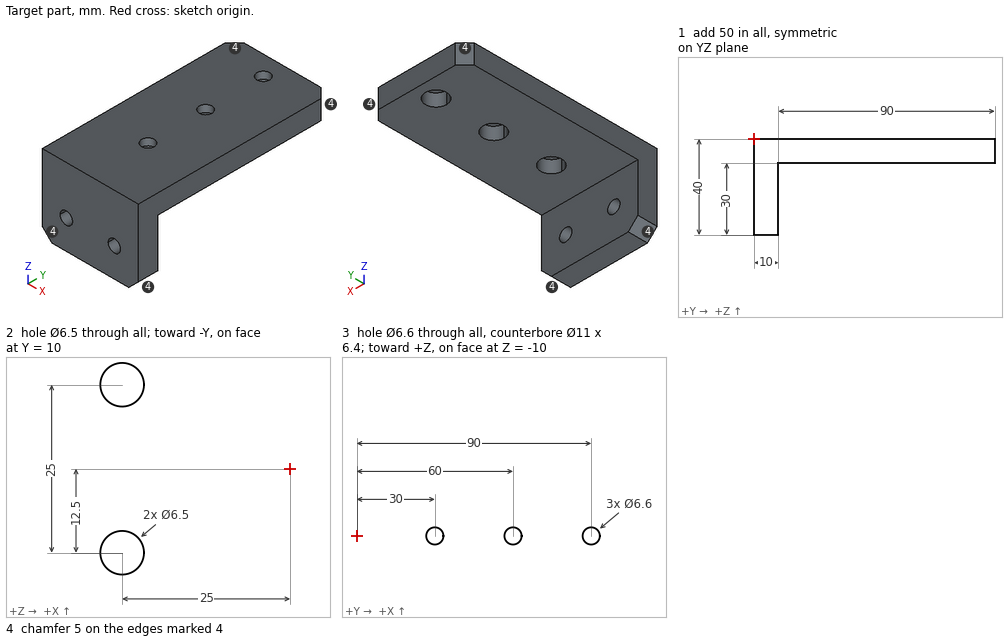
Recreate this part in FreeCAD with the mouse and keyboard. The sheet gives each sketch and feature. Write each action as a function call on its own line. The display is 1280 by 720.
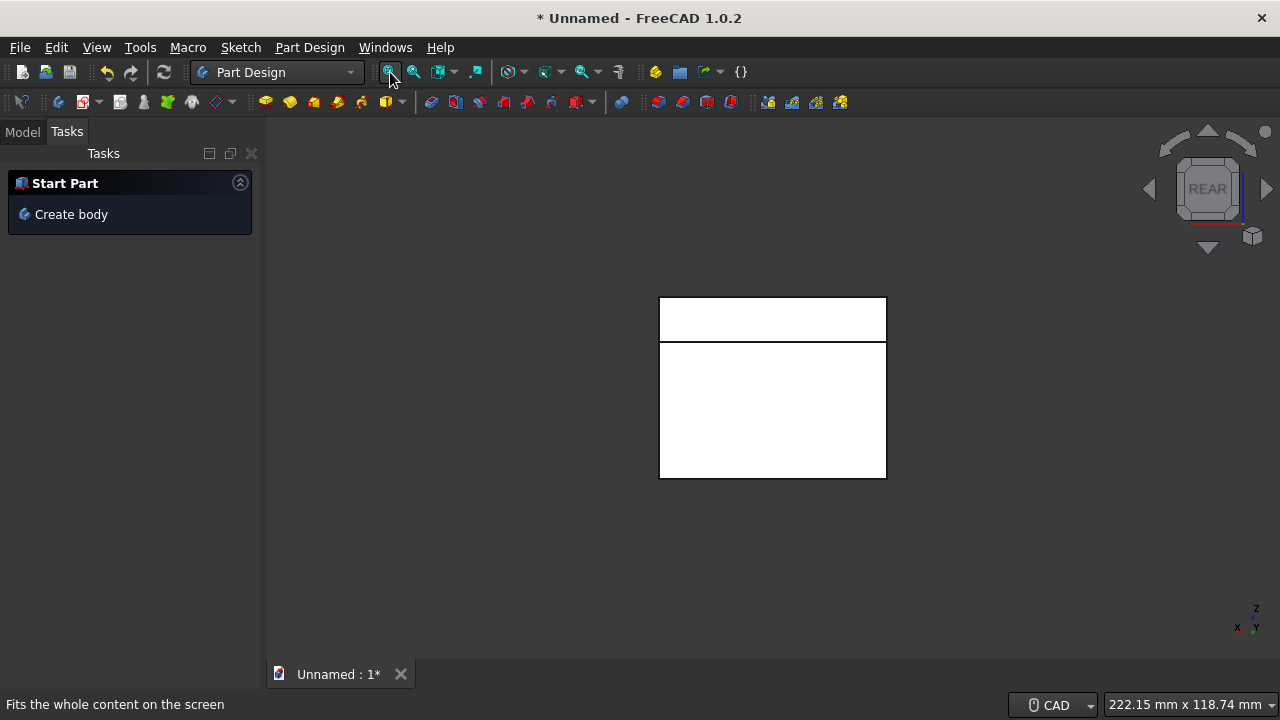
click(806, 410)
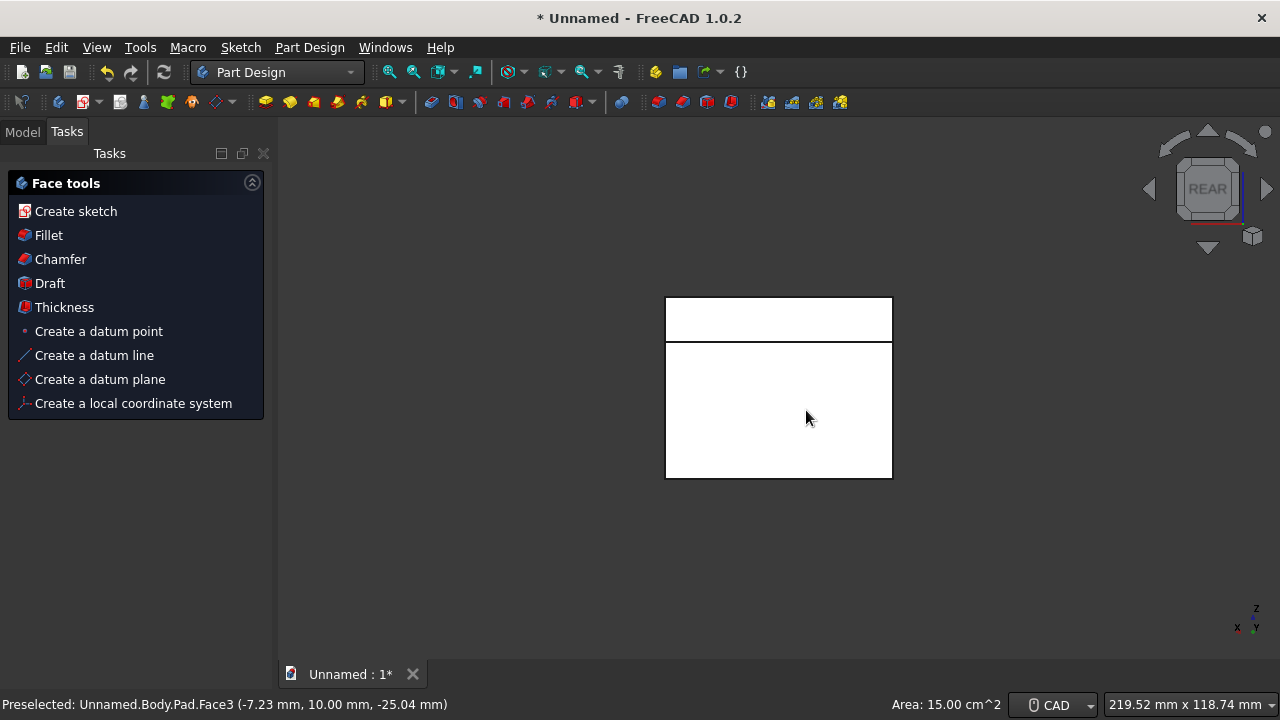
click(84, 102)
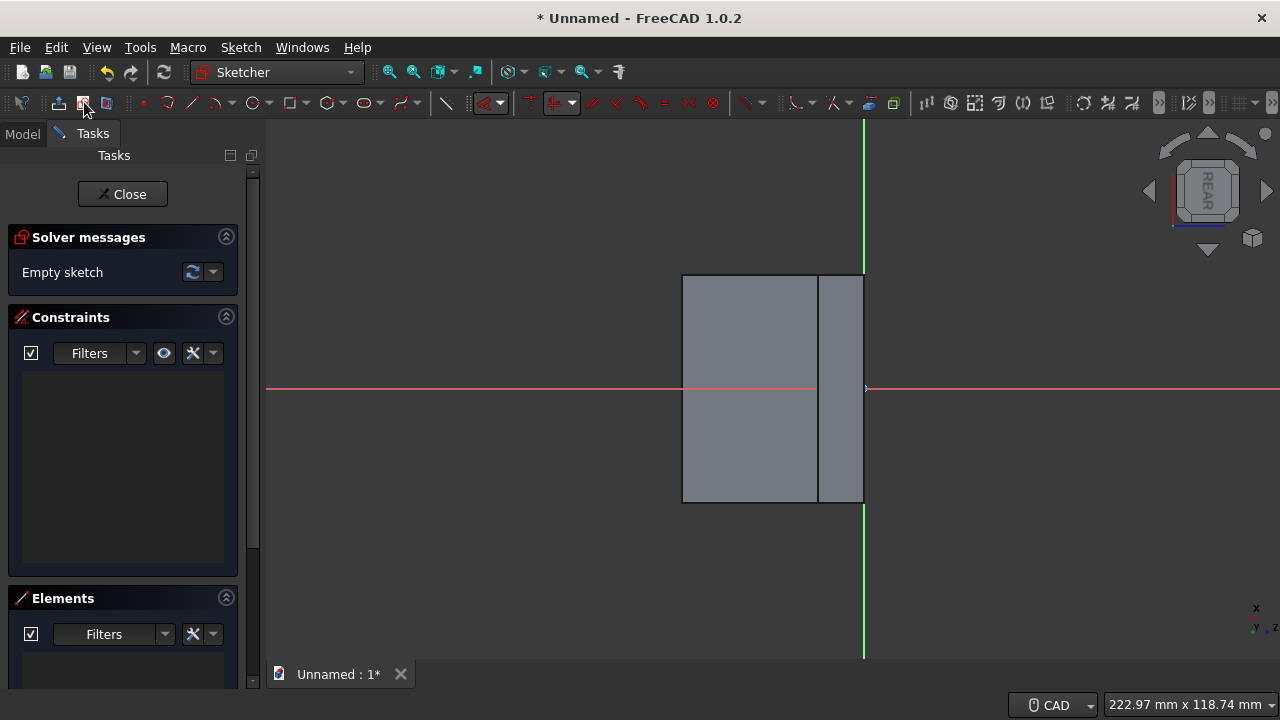
scroll(877, 389, up, 4)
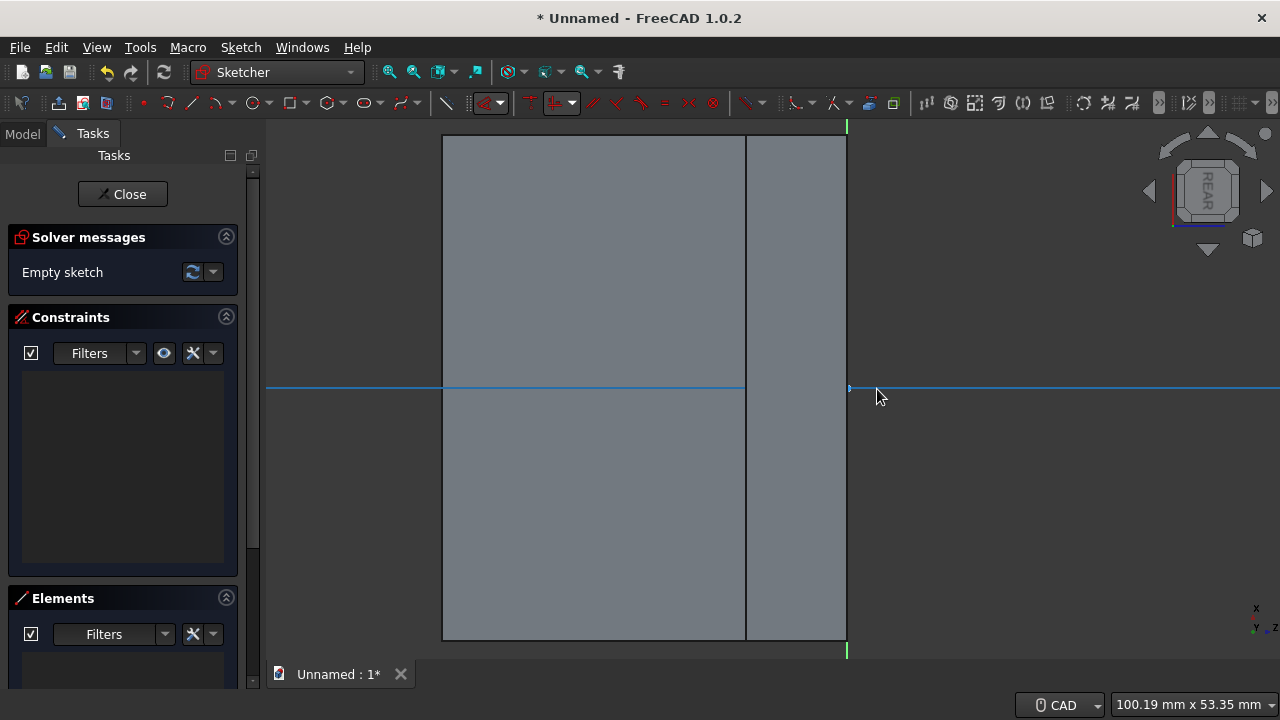
click(254, 104)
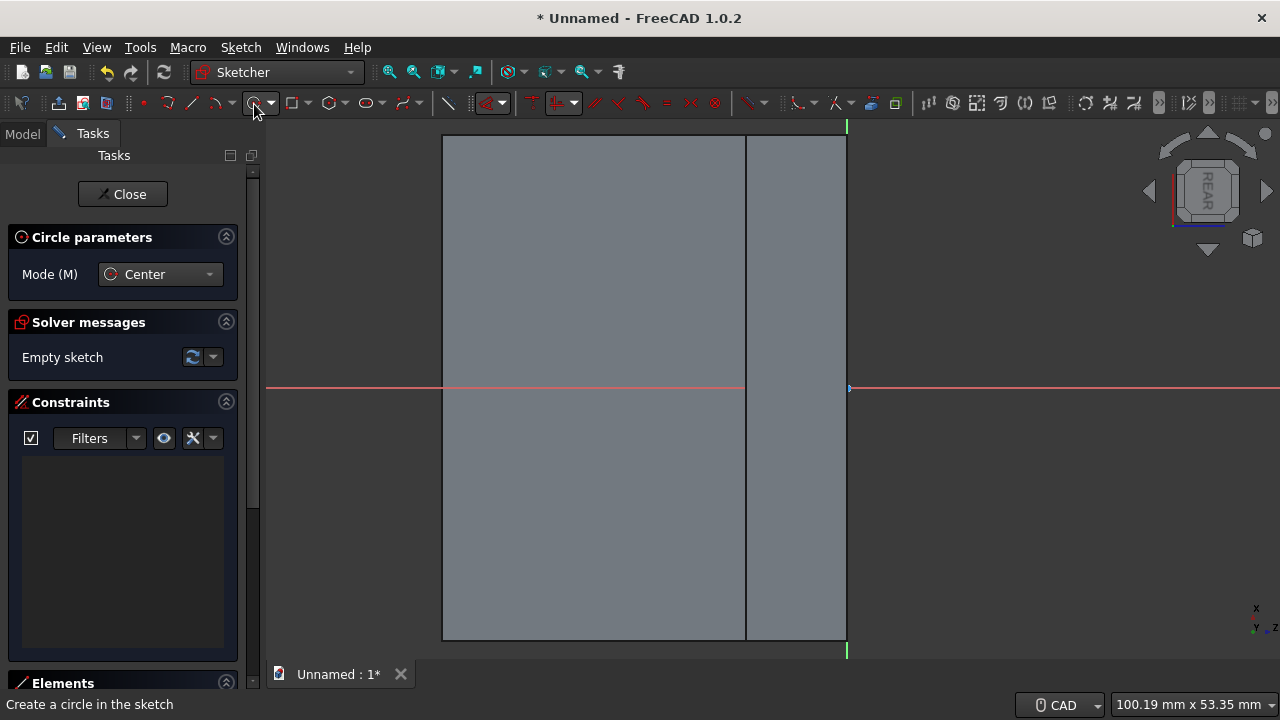
click(594, 515)
click(617, 492)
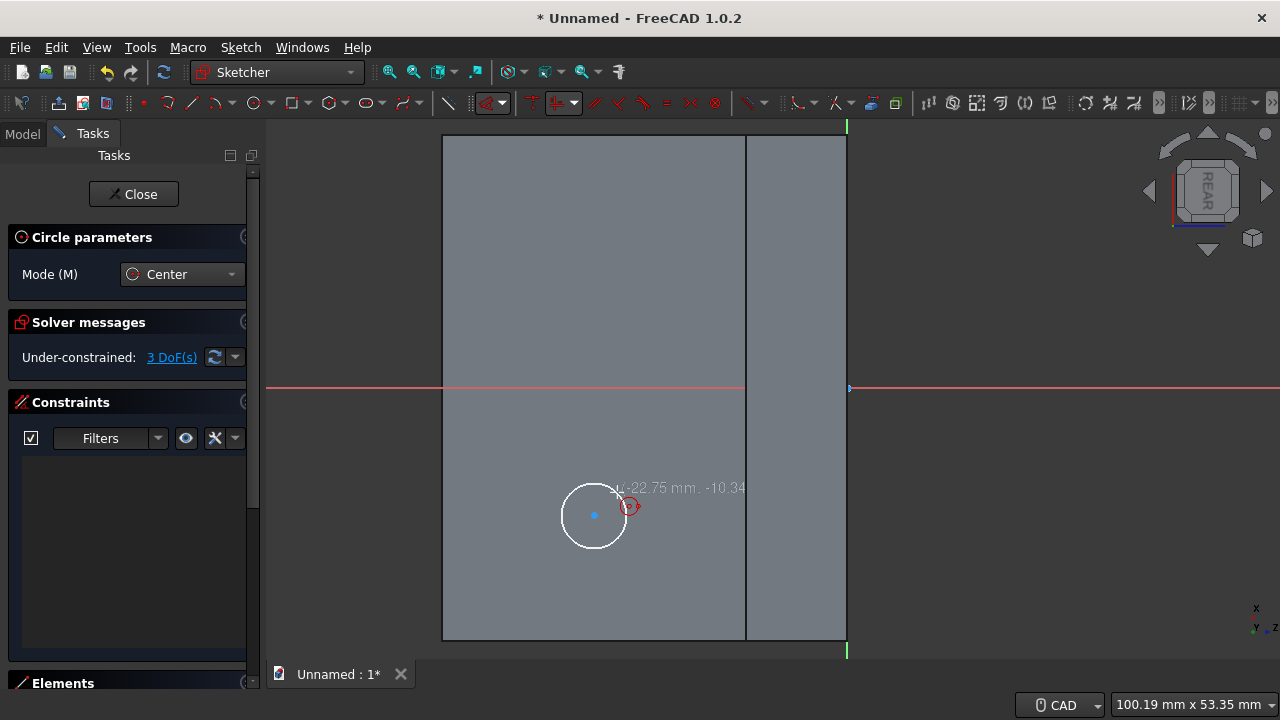
click(594, 262)
click(617, 239)
key(Escape)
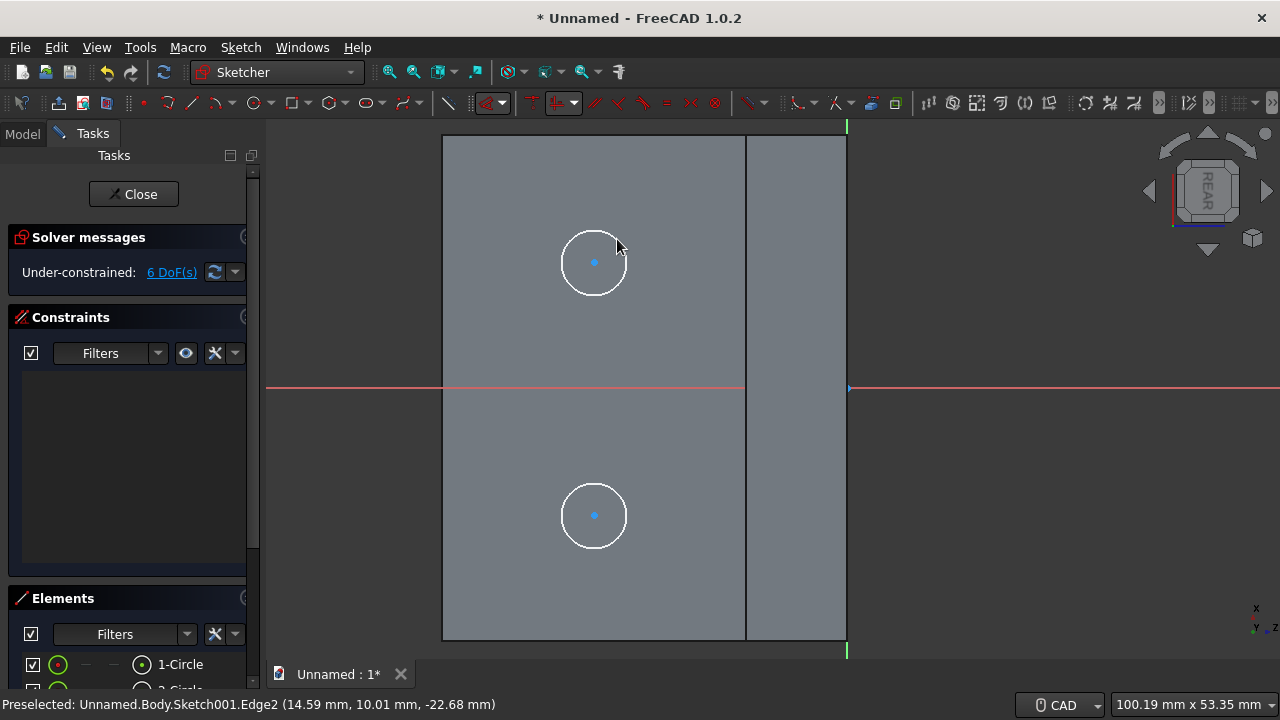
click(617, 493)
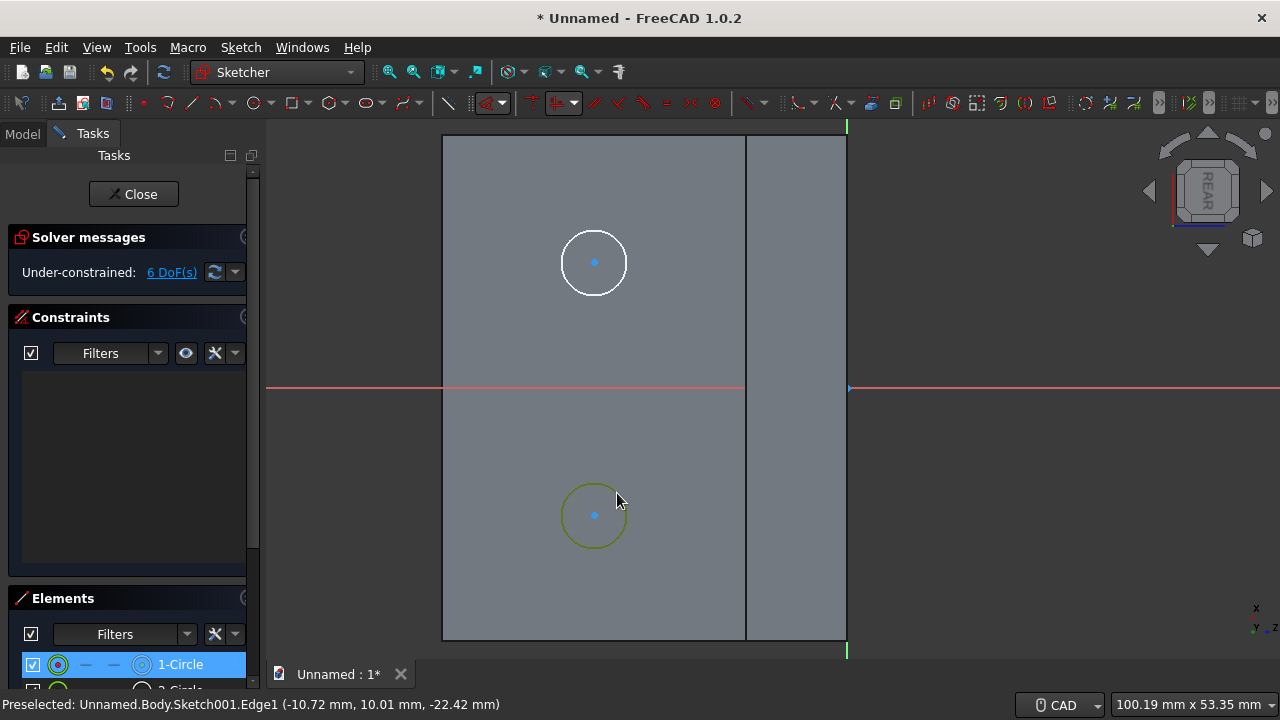
click(617, 240)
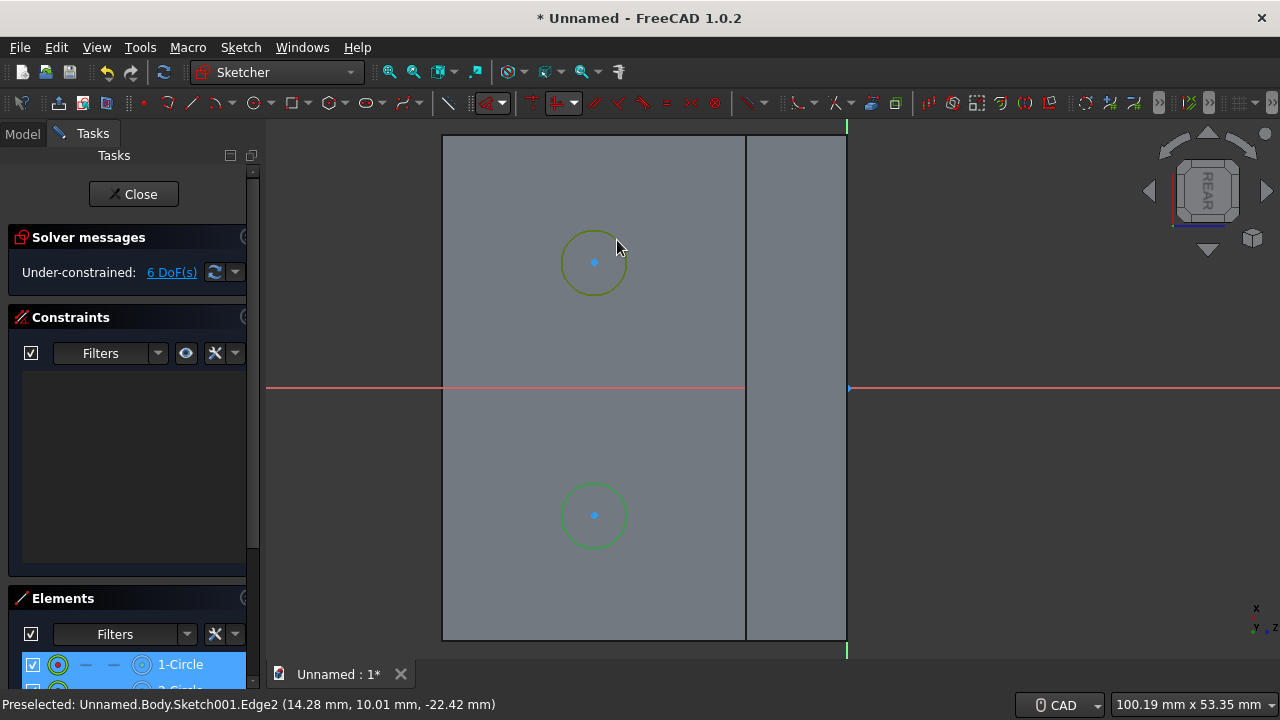
click(668, 104)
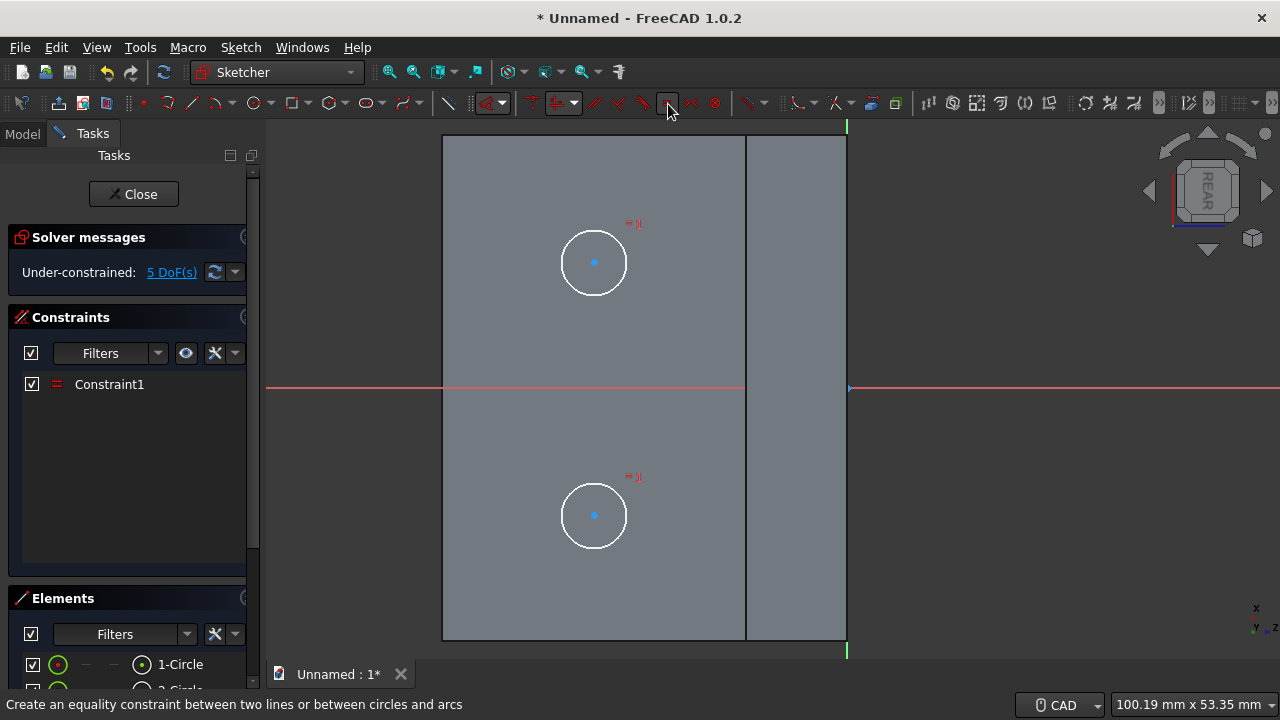
click(594, 516)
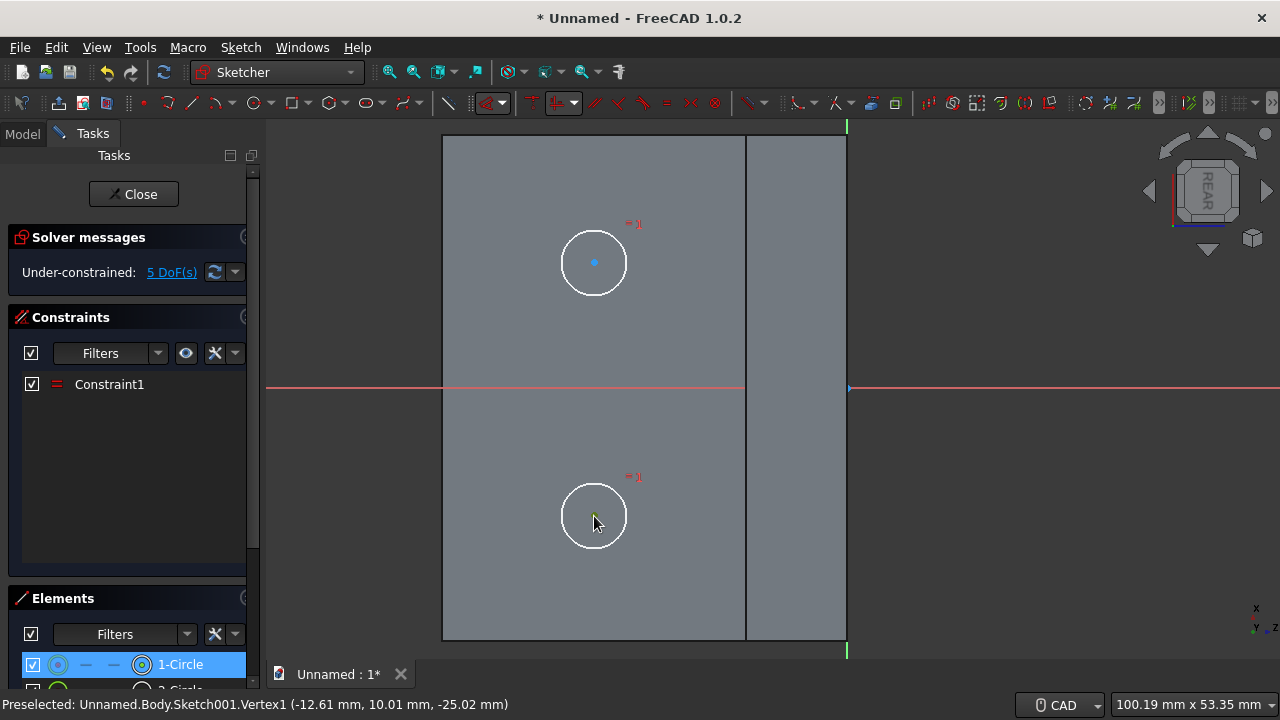
click(594, 263)